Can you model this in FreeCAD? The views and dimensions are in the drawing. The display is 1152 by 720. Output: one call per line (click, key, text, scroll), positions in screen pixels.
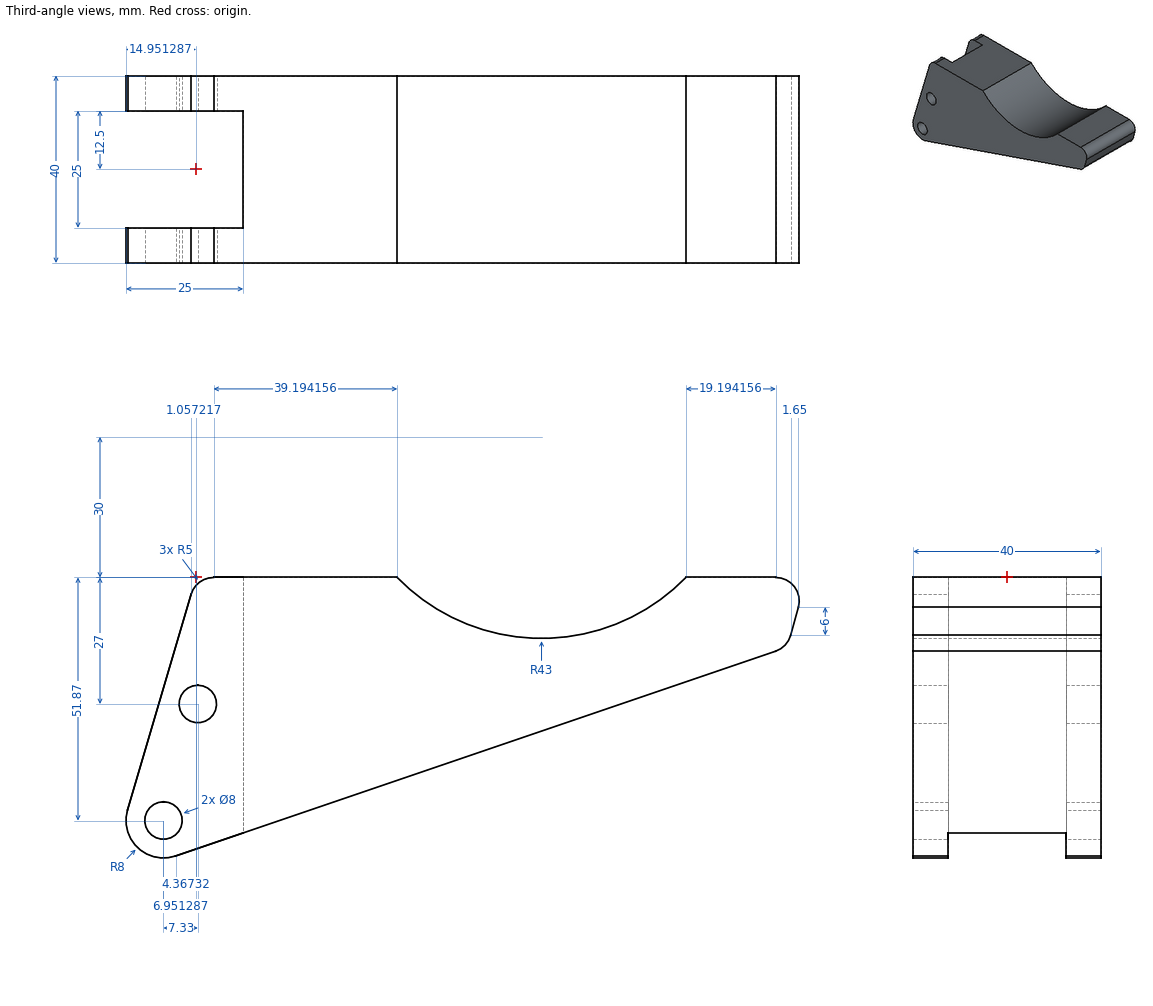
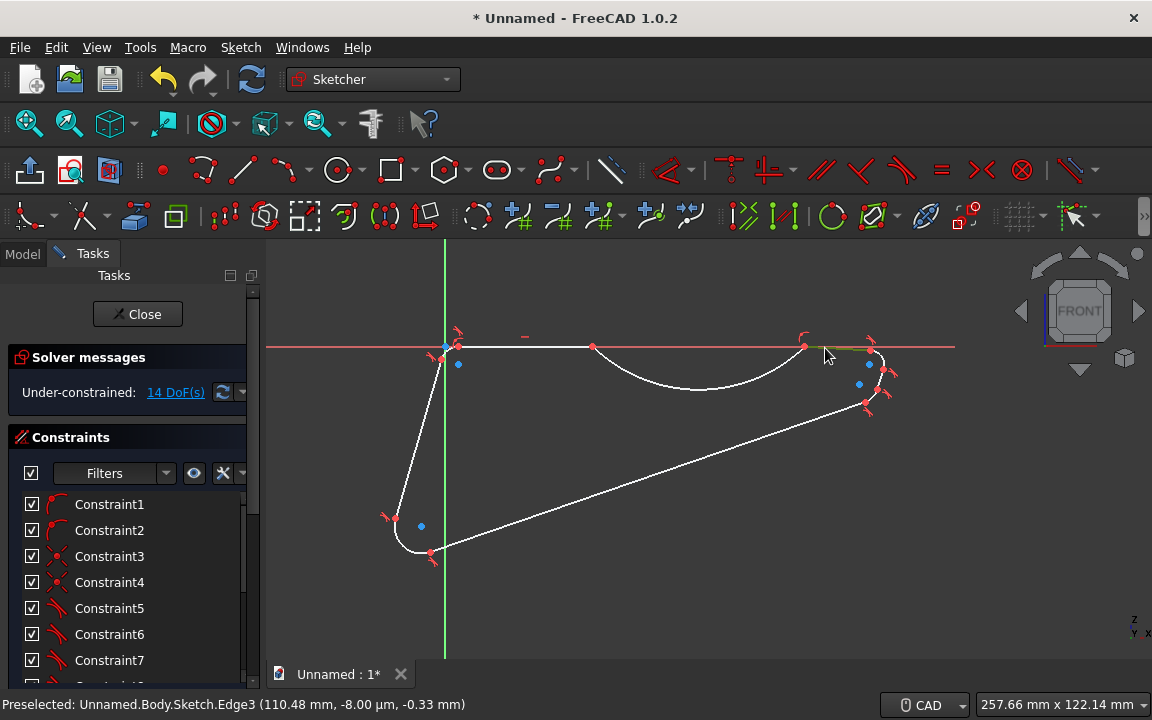
click(796, 170)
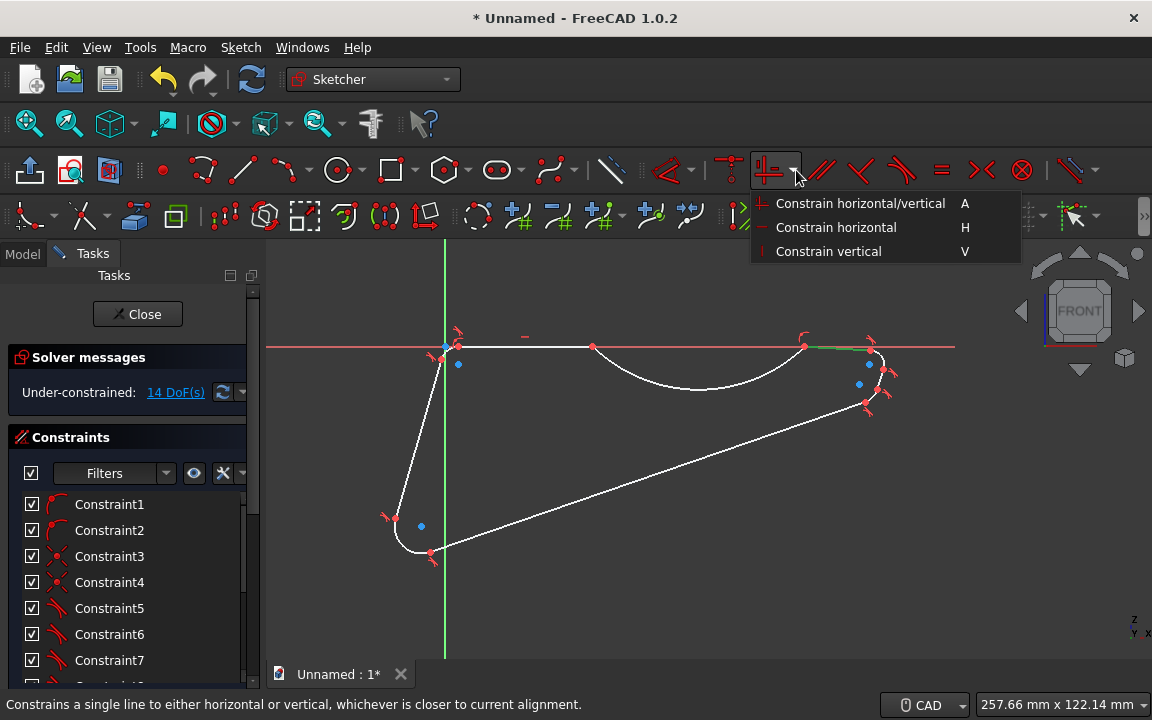
click(886, 227)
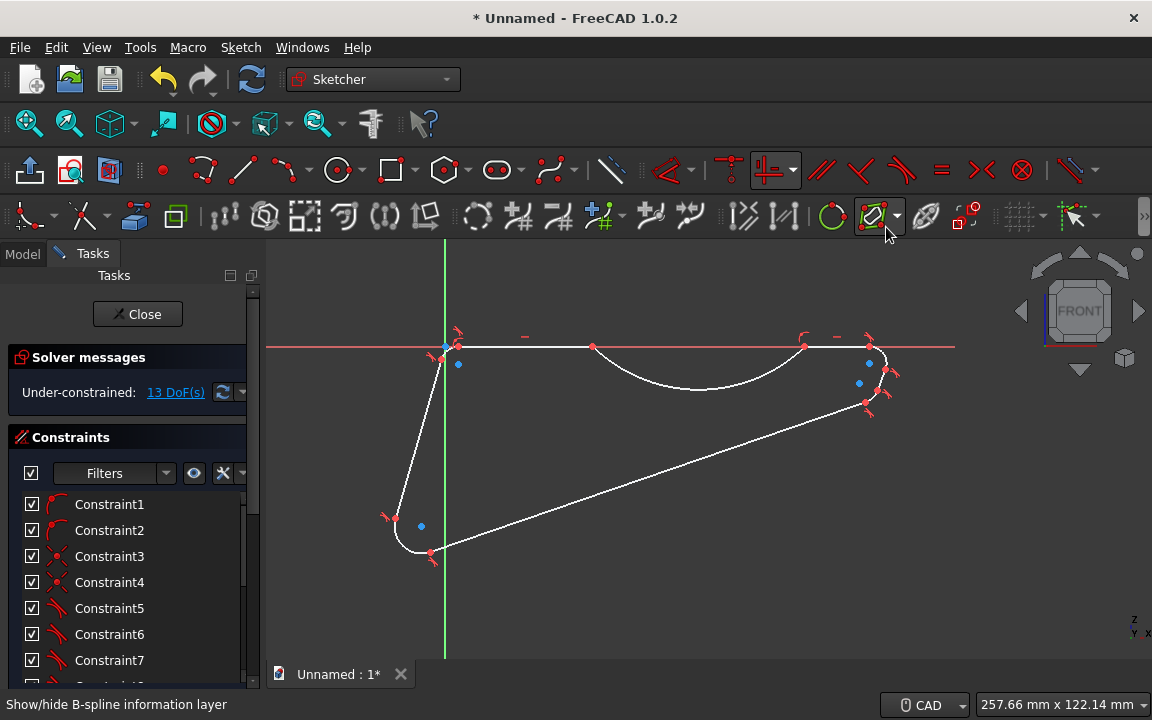
scroll(448, 350, up, 2)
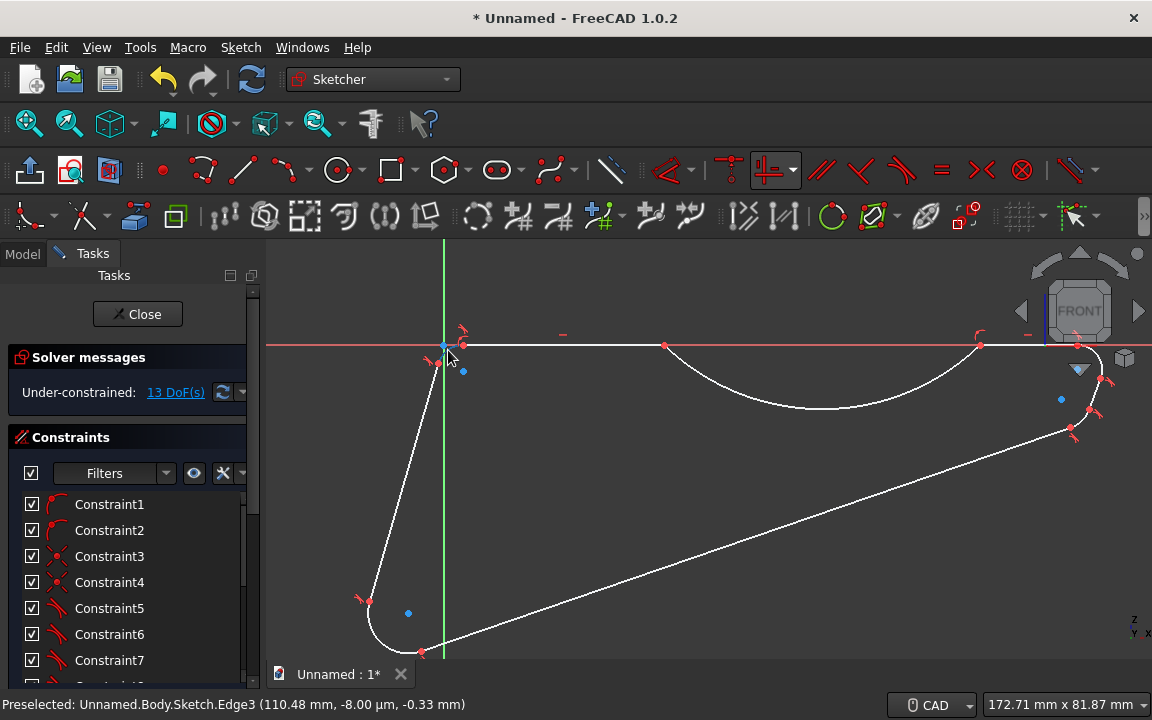
click(448, 350)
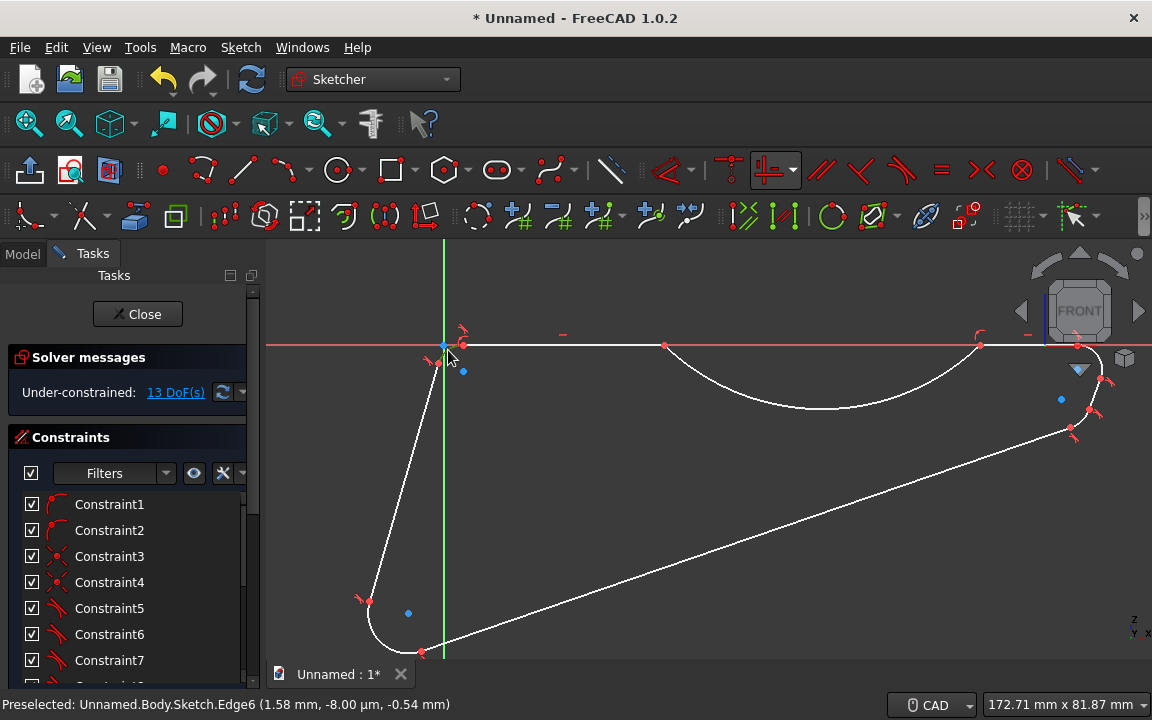
scroll(447, 350, down, 2)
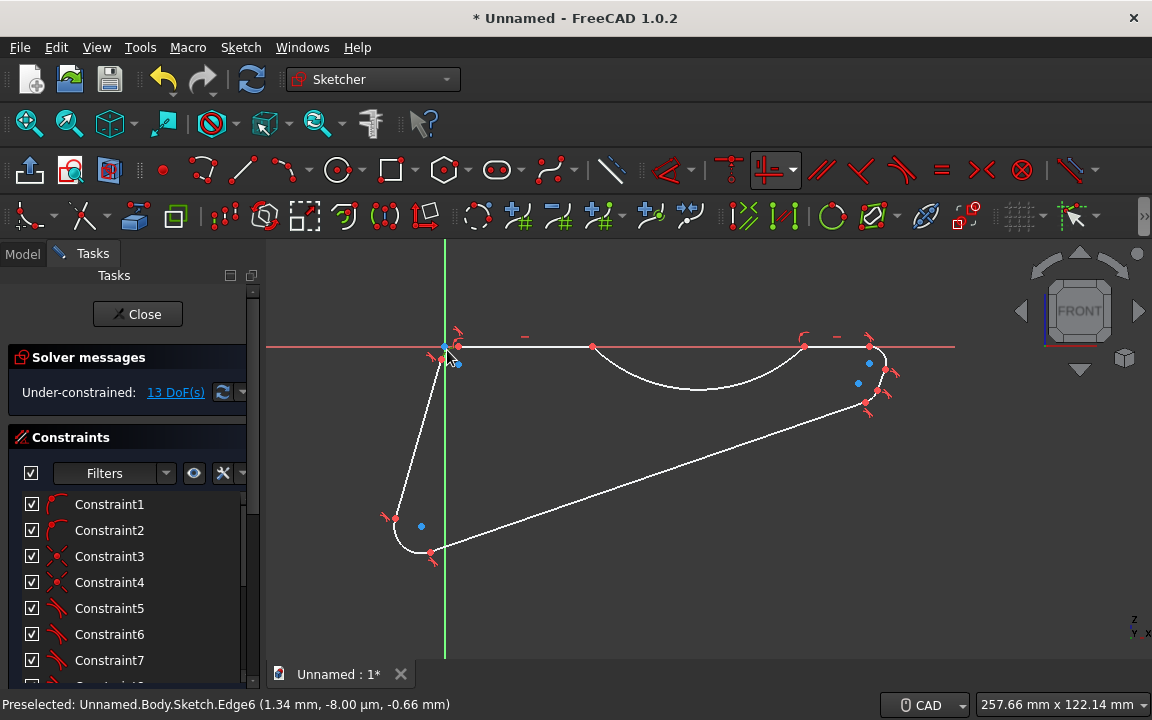
scroll(886, 360, up, 2)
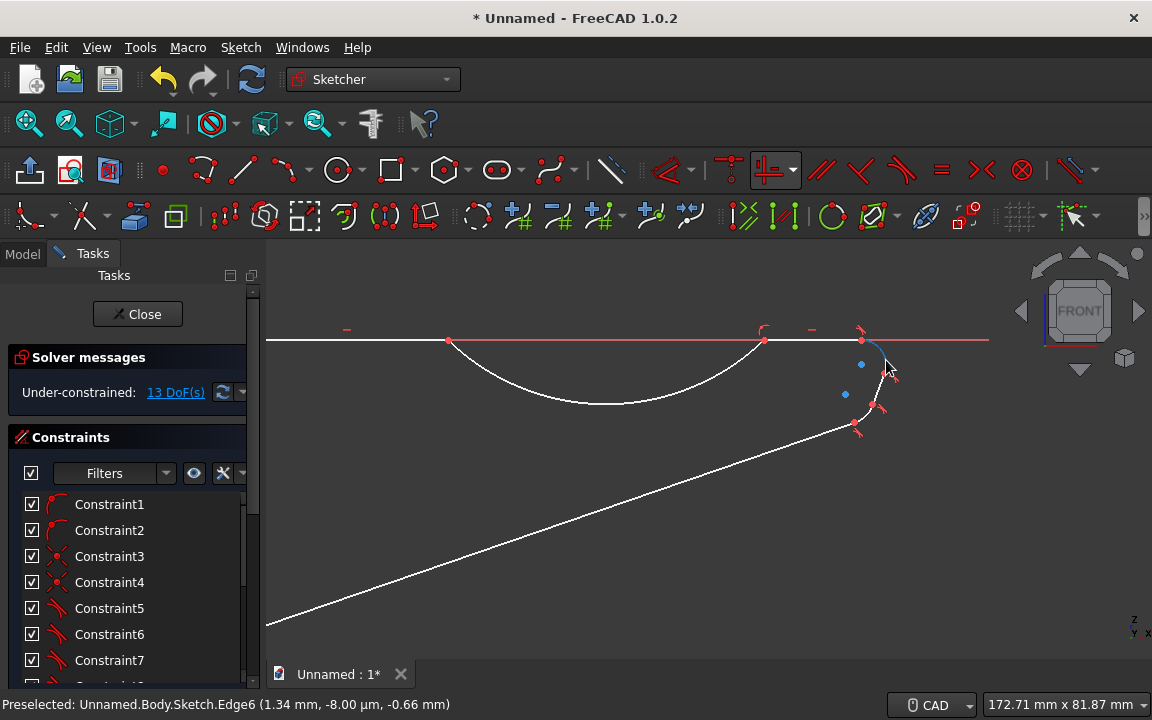
click(885, 359)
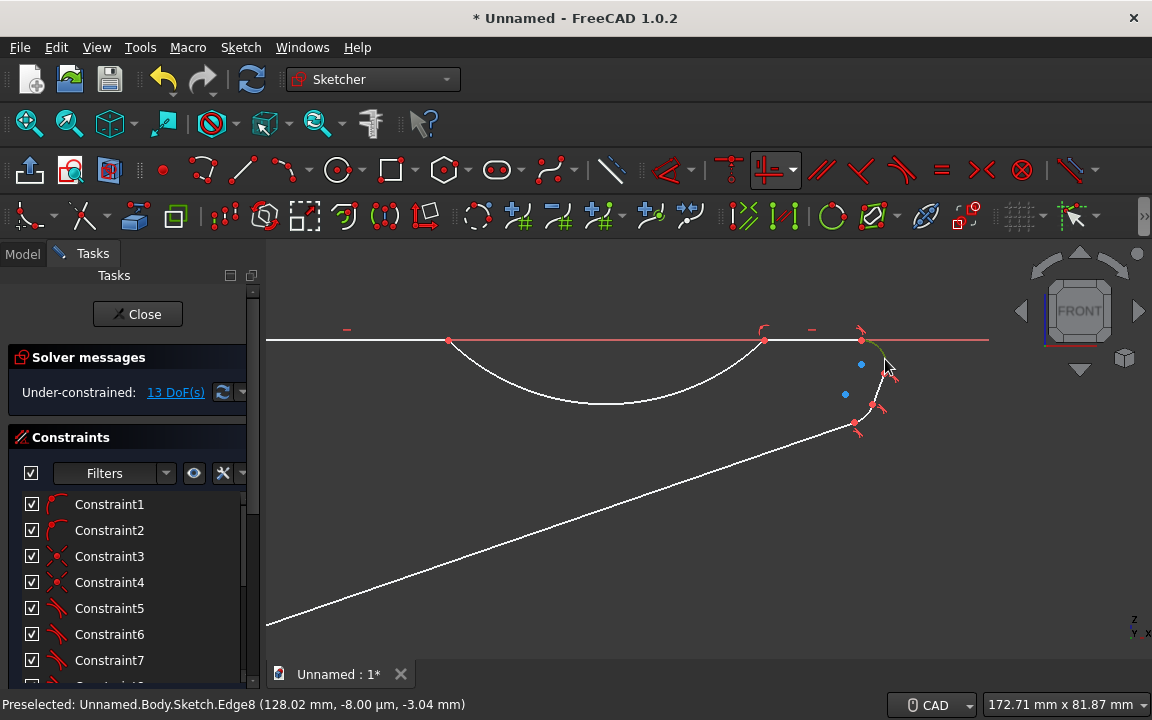
click(866, 416)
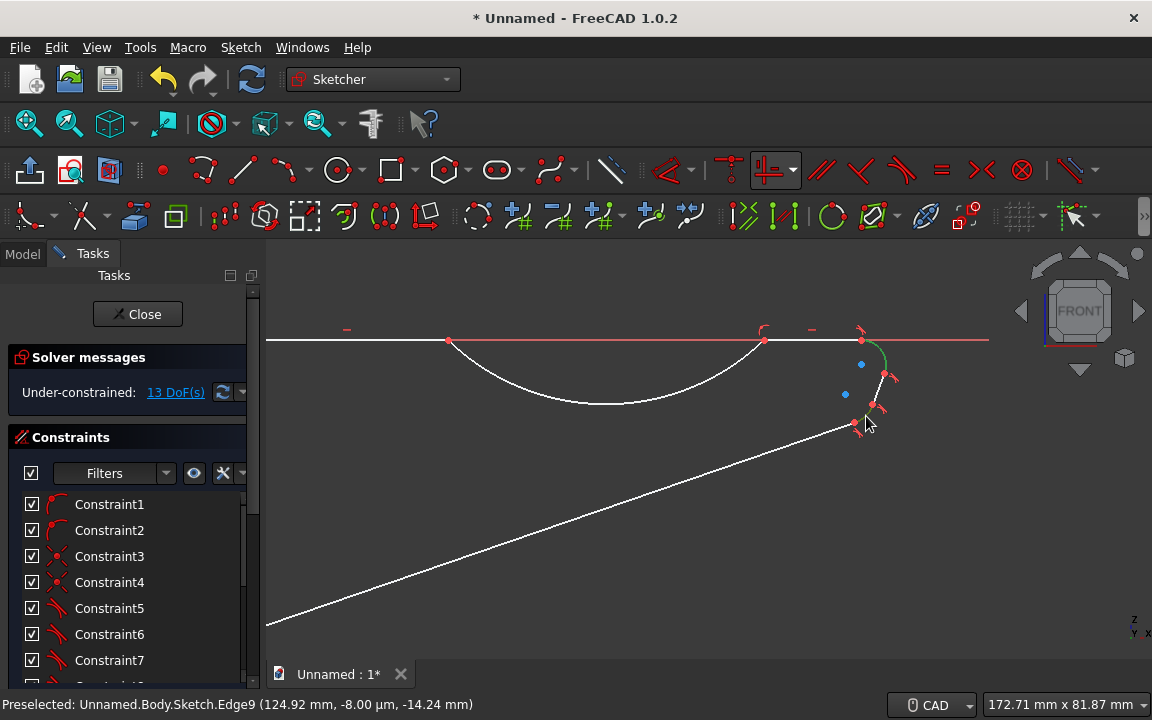
click(942, 170)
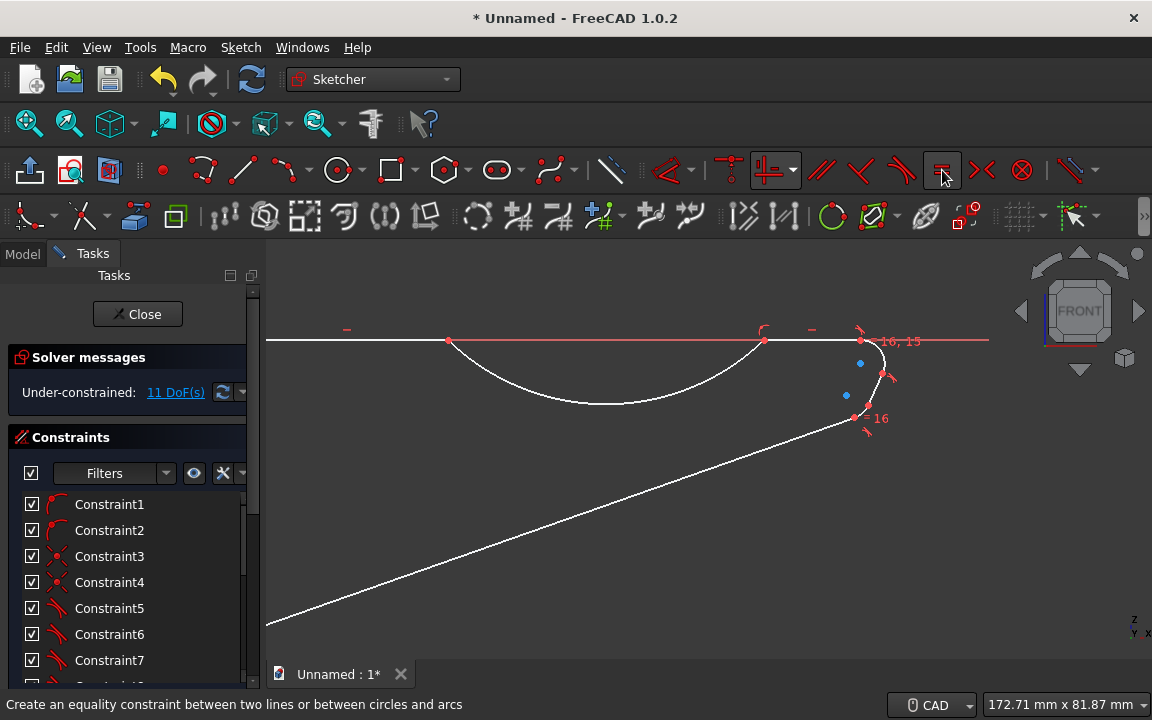
click(666, 170)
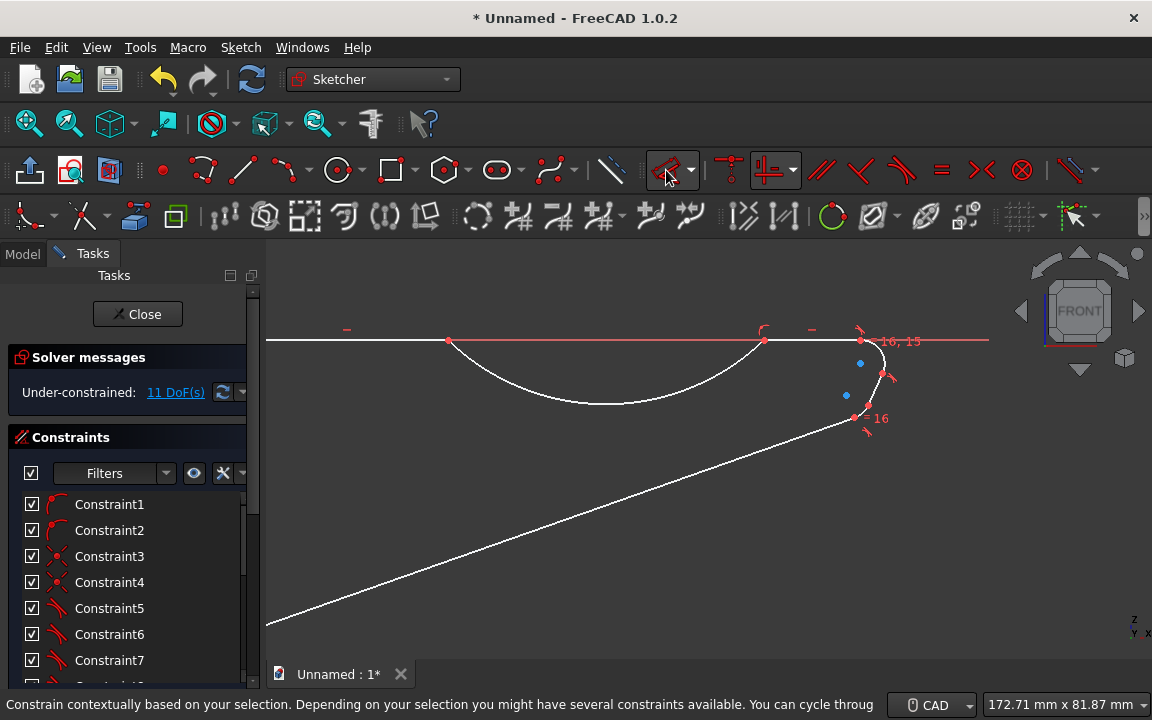
scroll(886, 360, down, 2)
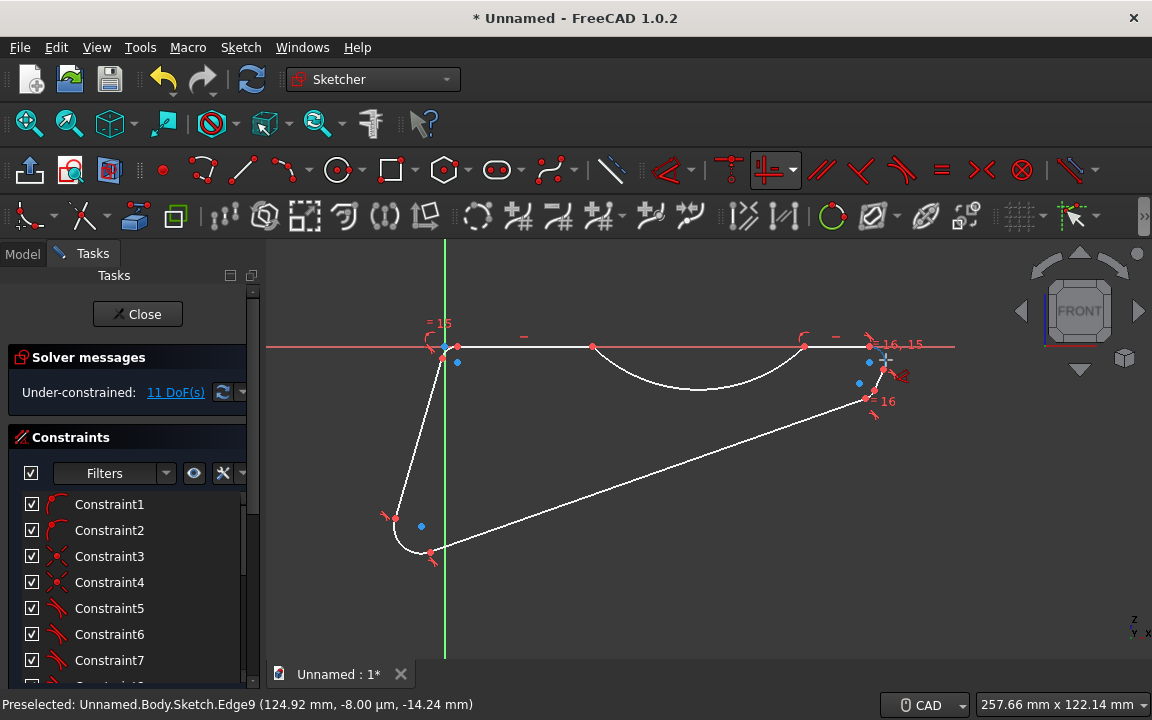
scroll(451, 348, up, 5)